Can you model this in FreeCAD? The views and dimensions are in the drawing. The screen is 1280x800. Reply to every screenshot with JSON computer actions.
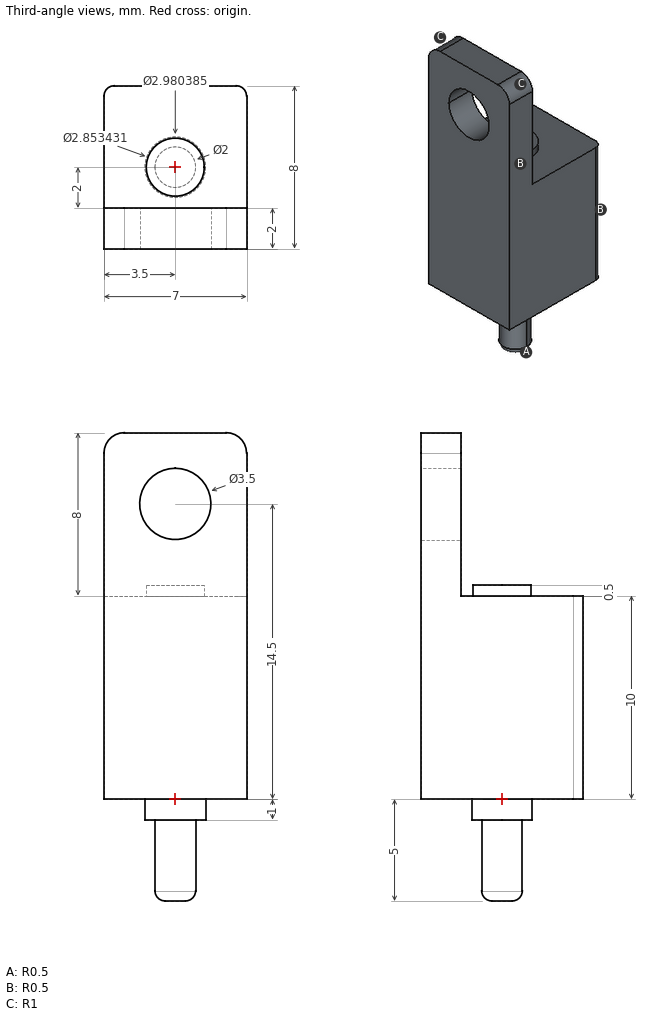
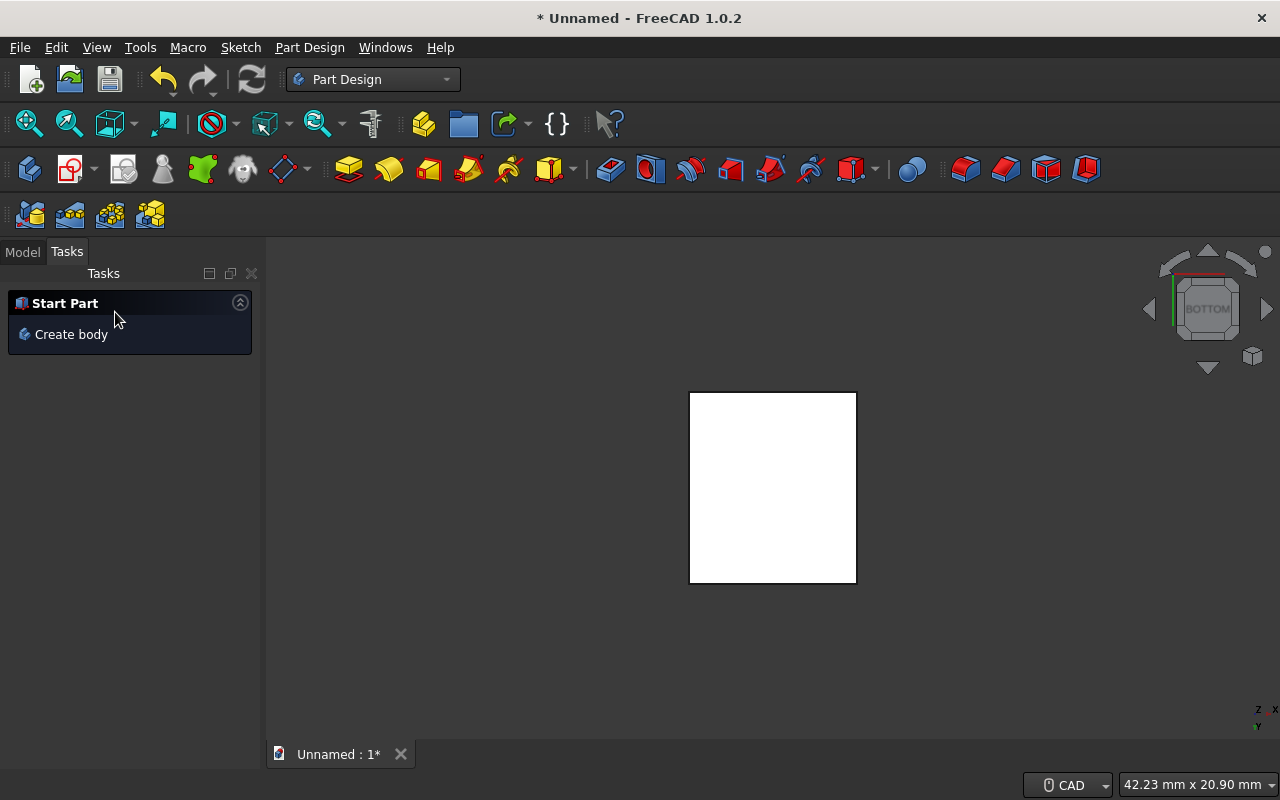
{"action": "key", "text": "v f"}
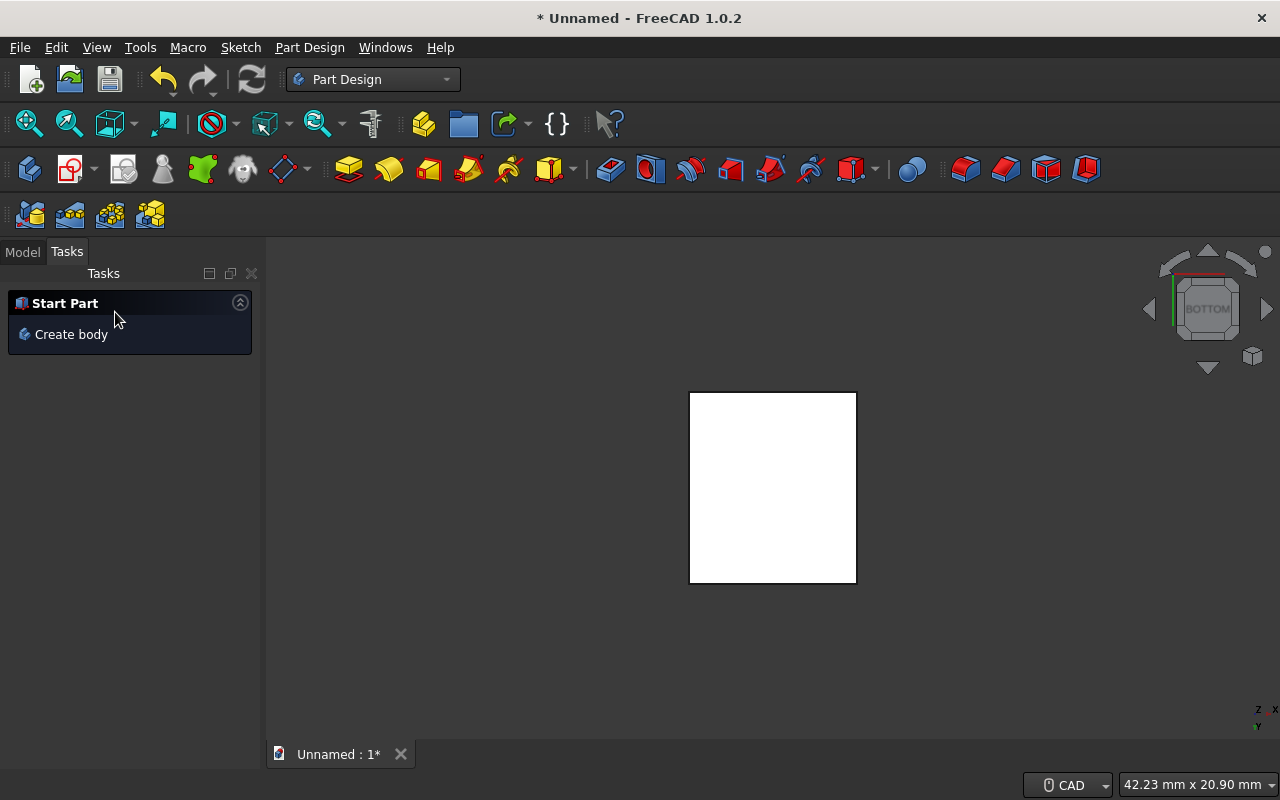
{"action": "left_click", "coordinate": [773, 487]}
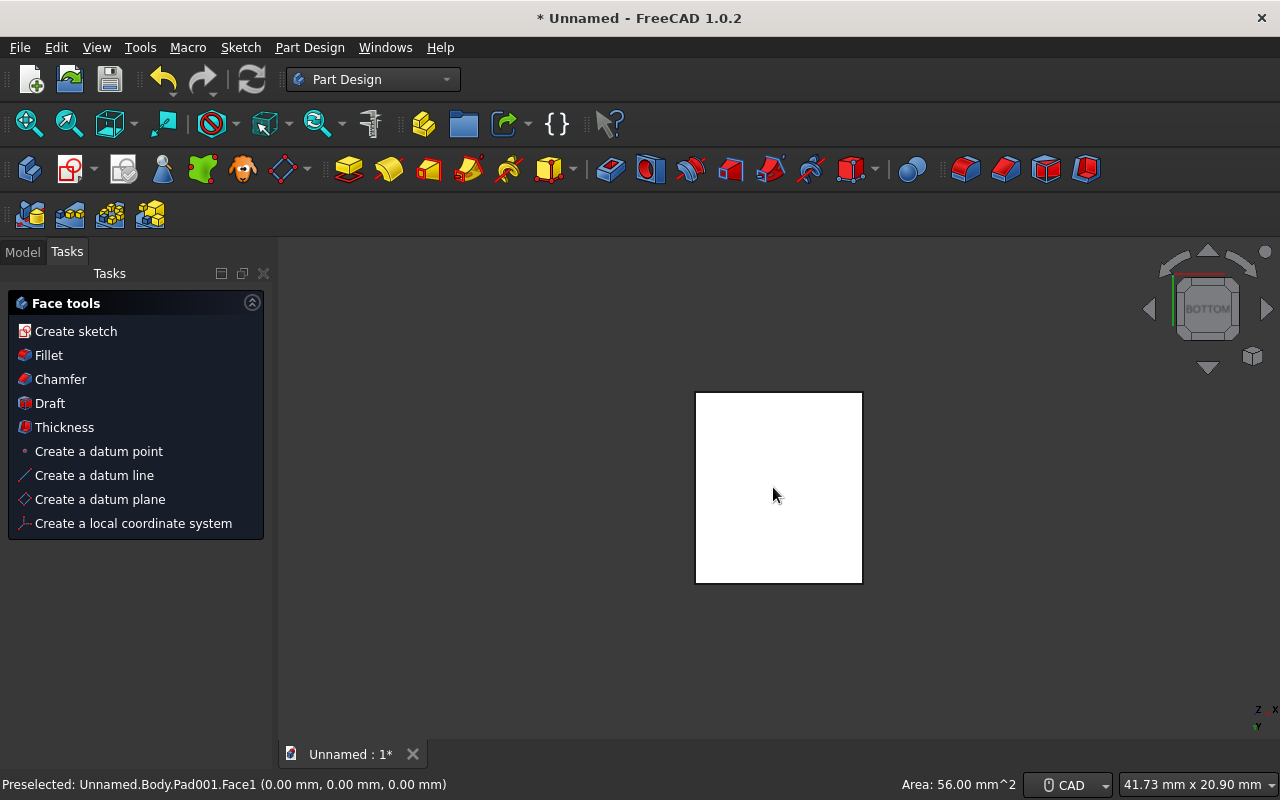
{"action": "left_click", "coordinate": [70, 170]}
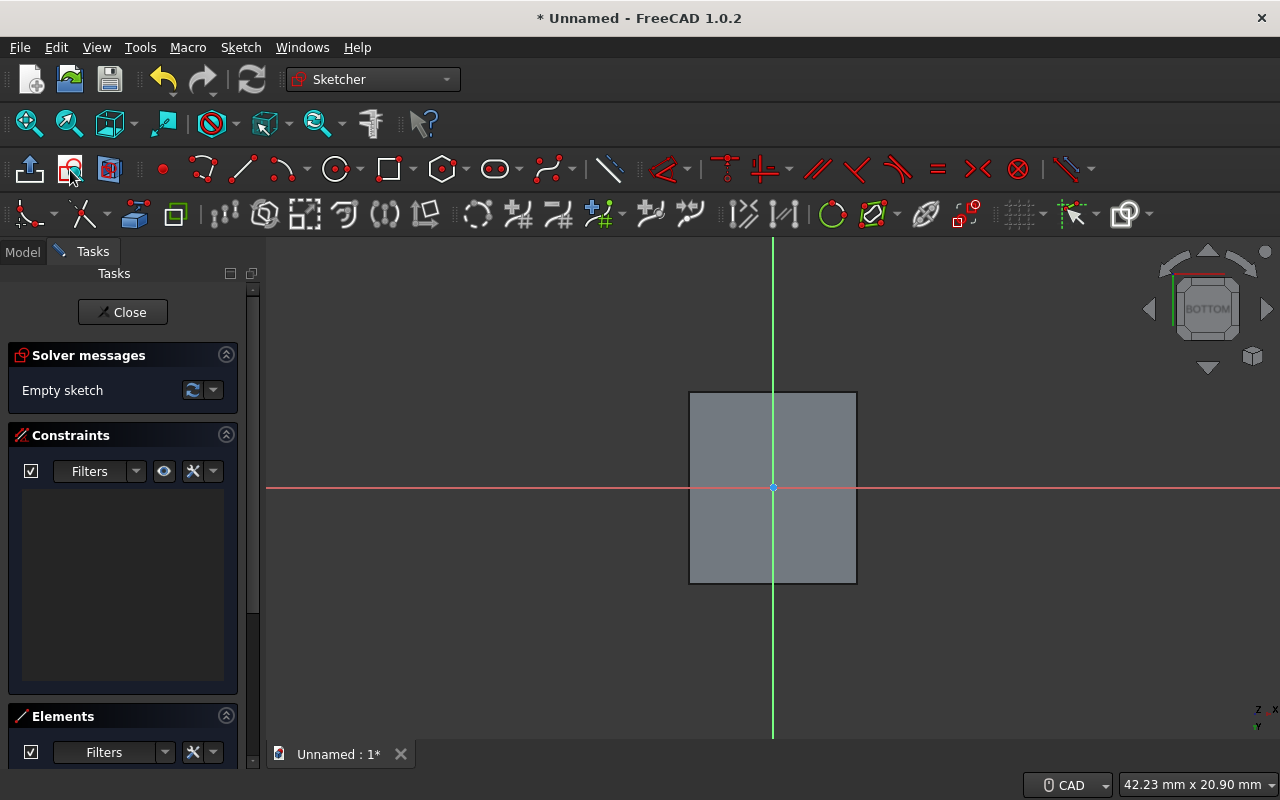
{"action": "scroll", "coordinate": [787, 488], "scroll_direction": "up", "scroll_amount": 9}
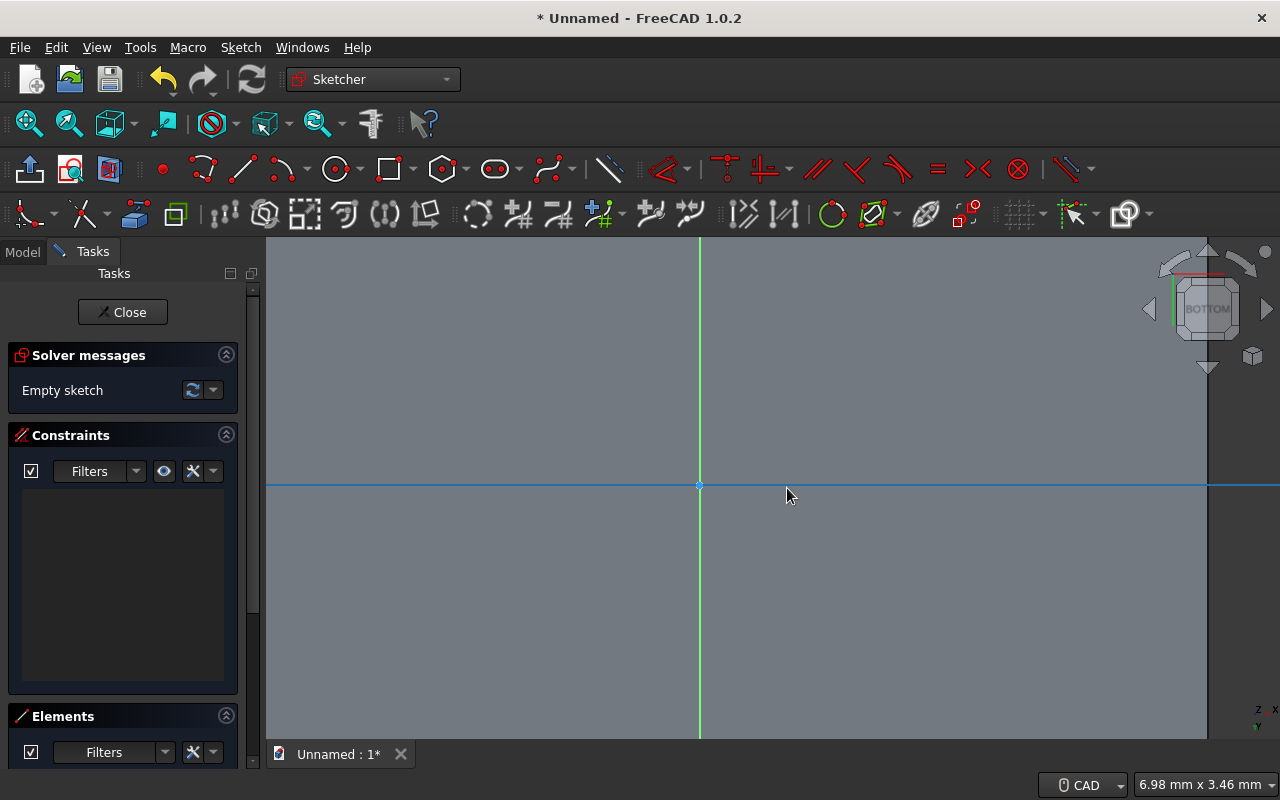
{"action": "key", "text": "g c"}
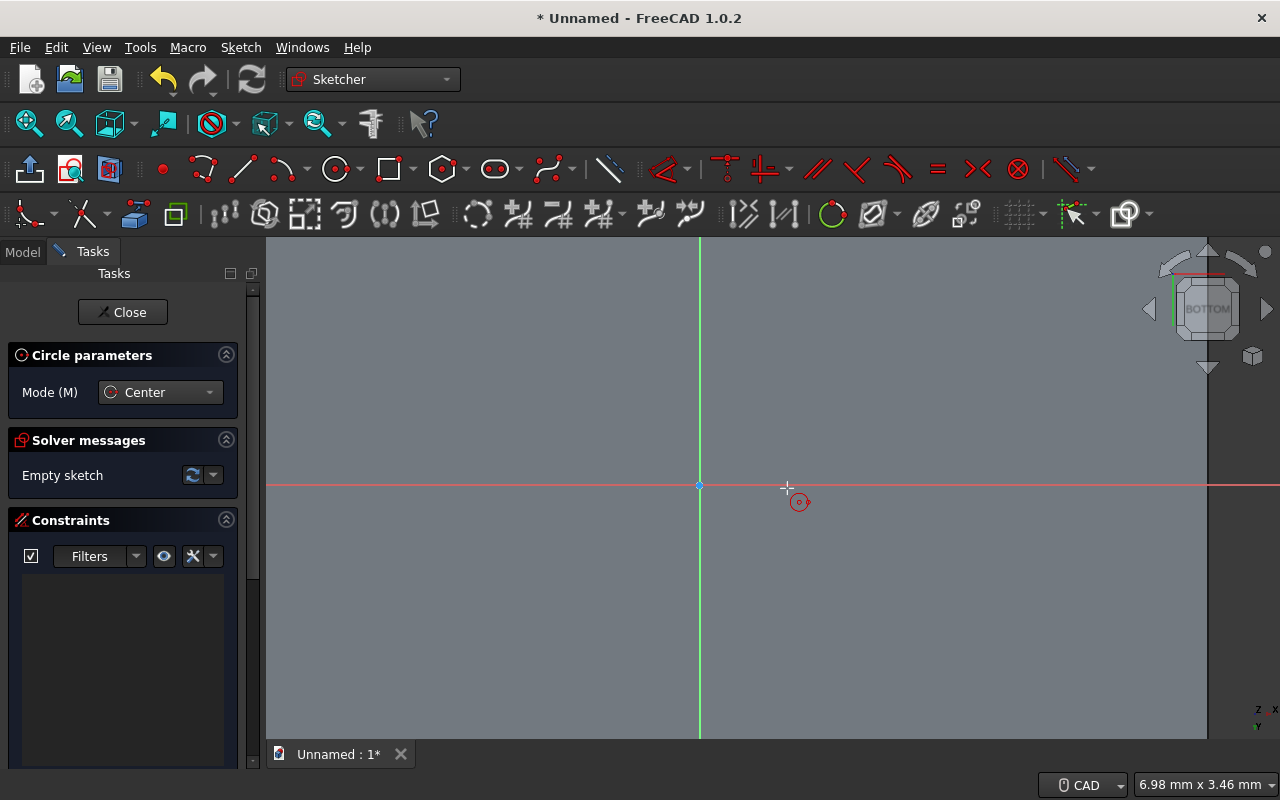
{"action": "left_click", "coordinate": [700, 485]}
{"action": "mouse_move", "coordinate": [802, 383]}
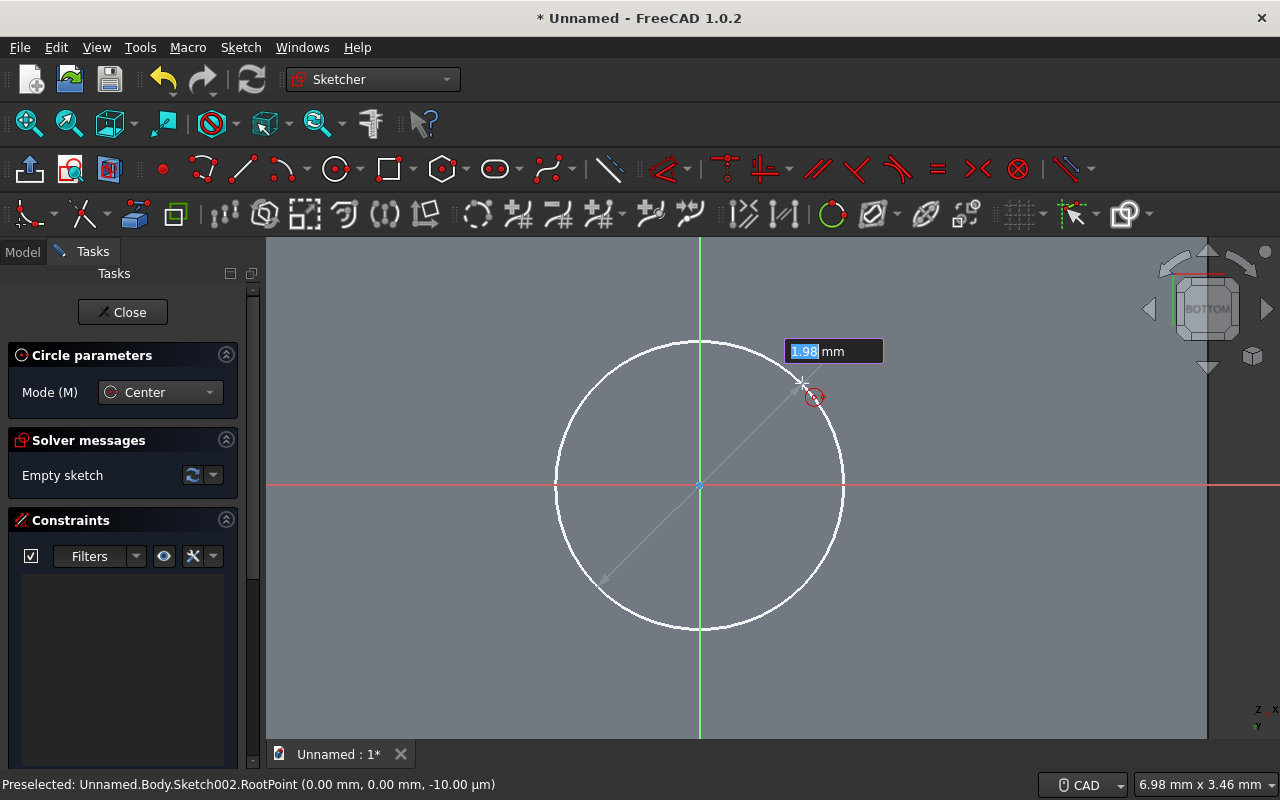
{"action": "type", "text": "2"}
{"action": "key", "text": "Return"}
{"action": "key", "text": "Escape"}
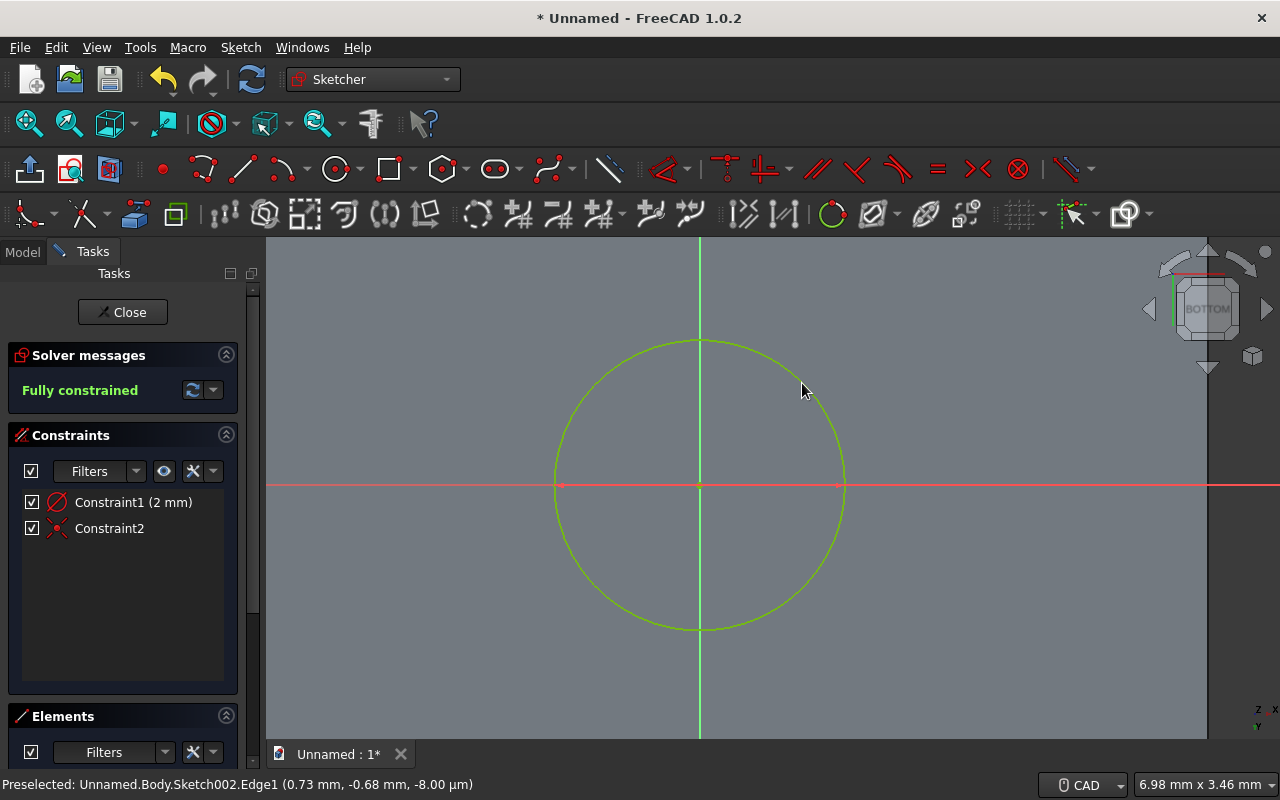
{"action": "left_click", "coordinate": [123, 312]}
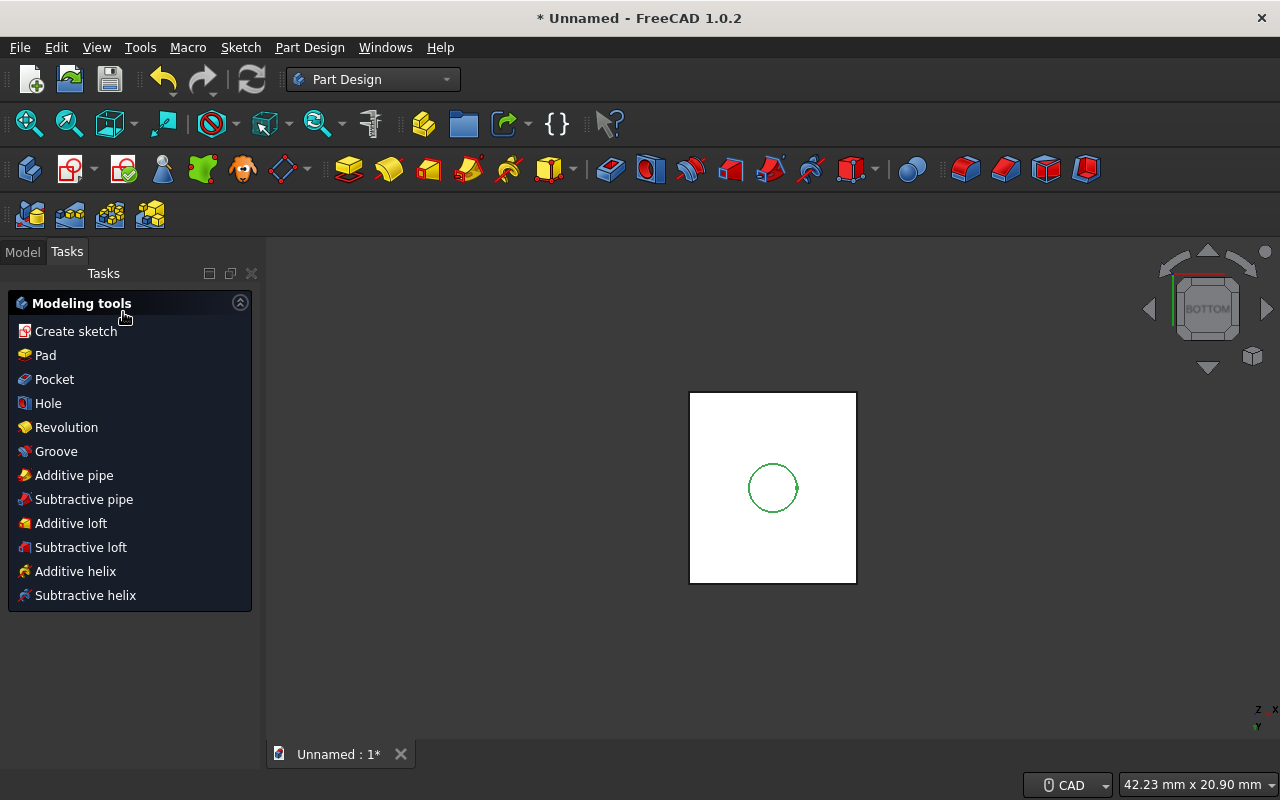
{"action": "left_click", "coordinate": [350, 170]}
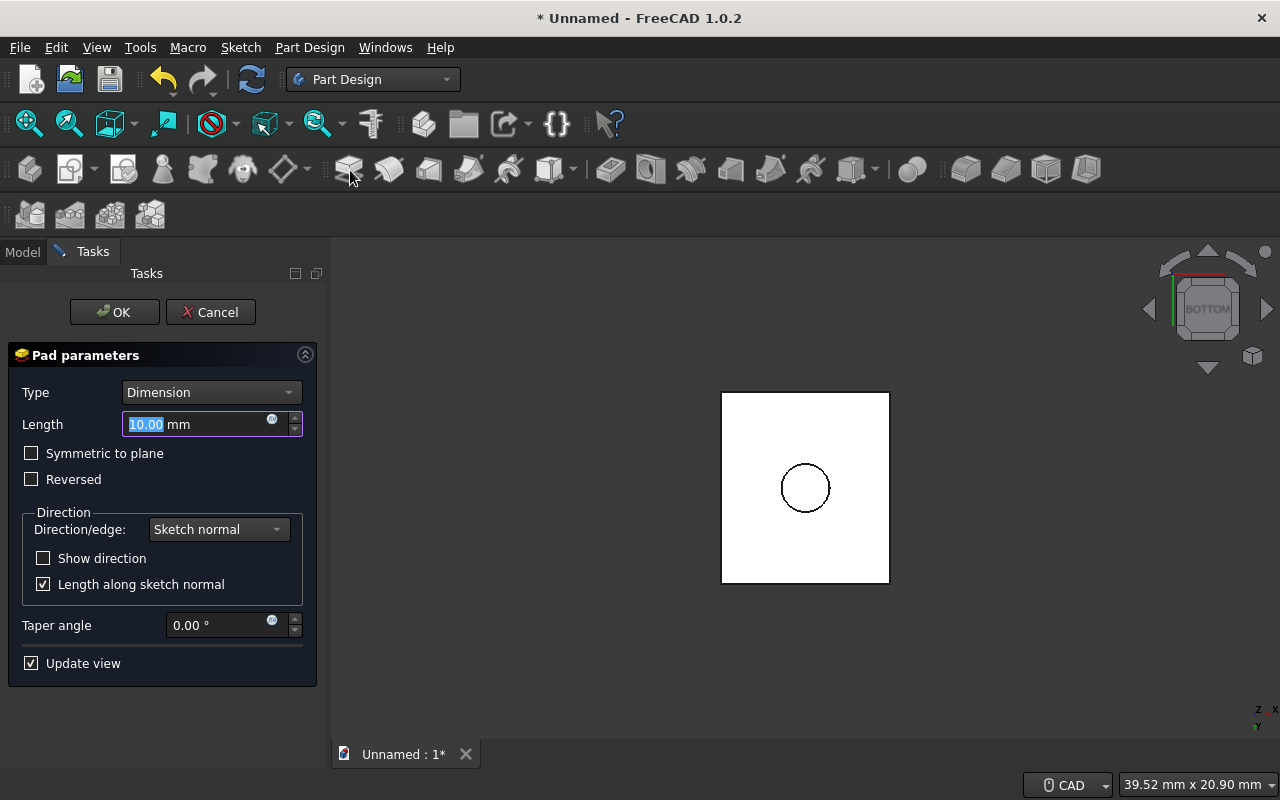
{"action": "type", "text": "5"}
{"action": "key", "text": "Tab"}